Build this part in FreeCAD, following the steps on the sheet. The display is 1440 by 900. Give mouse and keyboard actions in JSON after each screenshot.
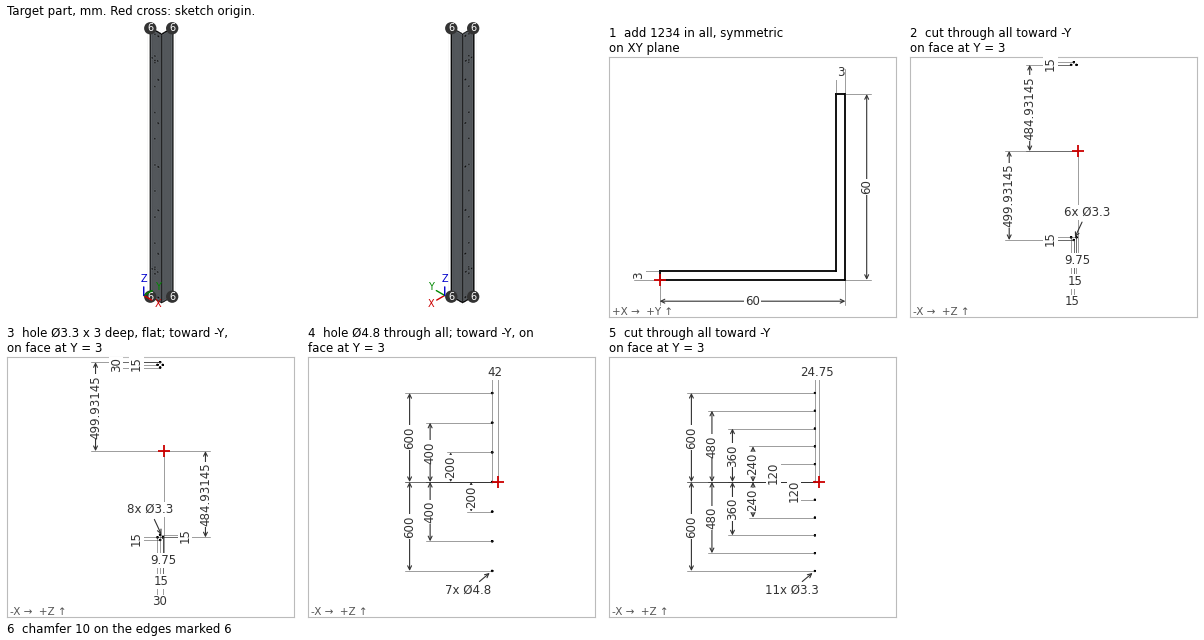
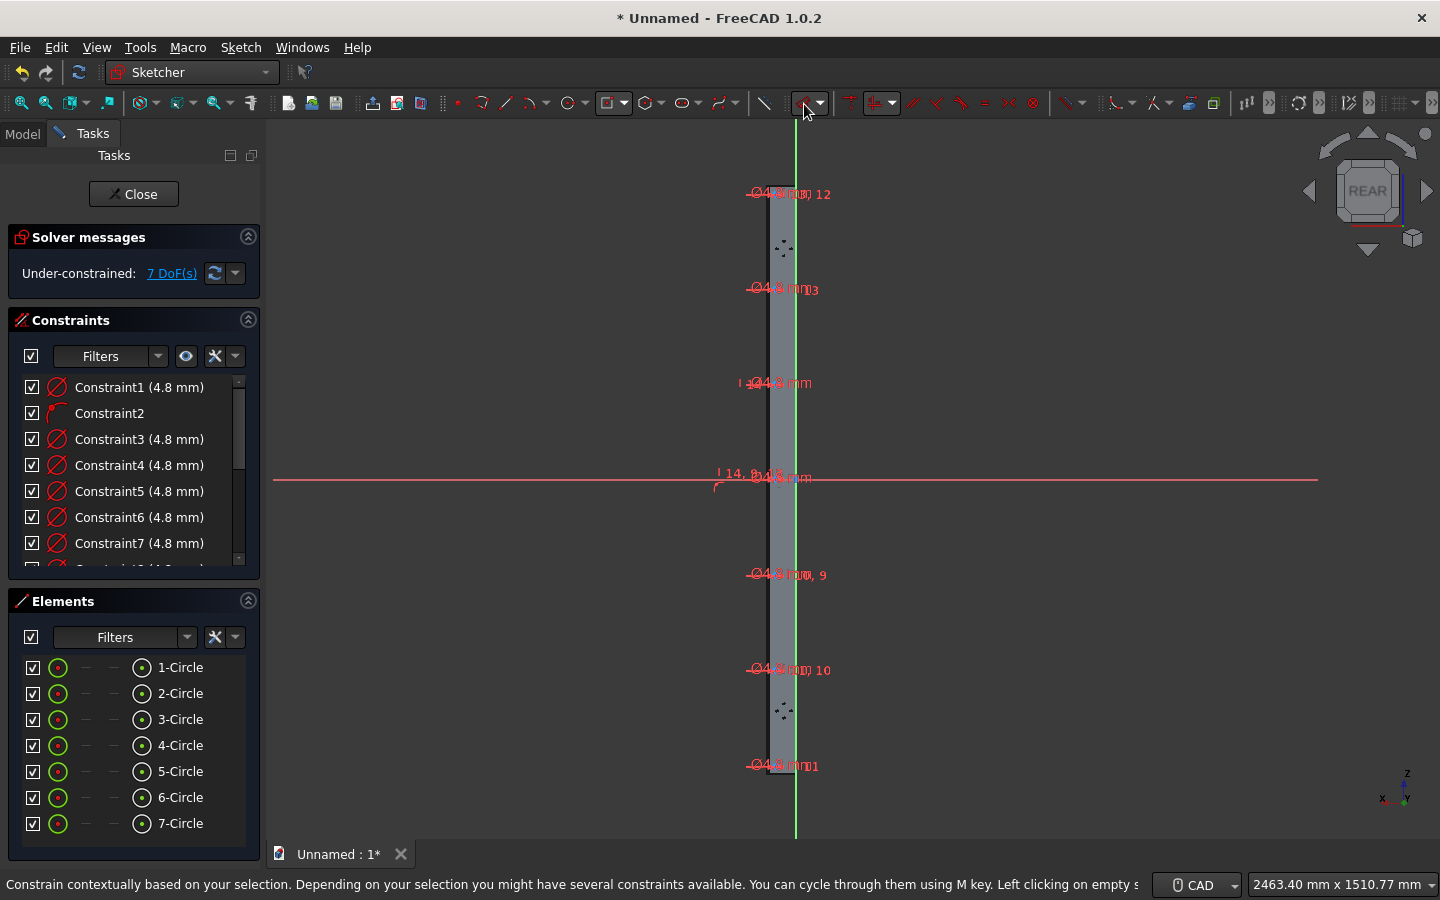
{"action": "scroll", "coordinate": [776, 480], "scroll_direction": "up", "scroll_amount": 4}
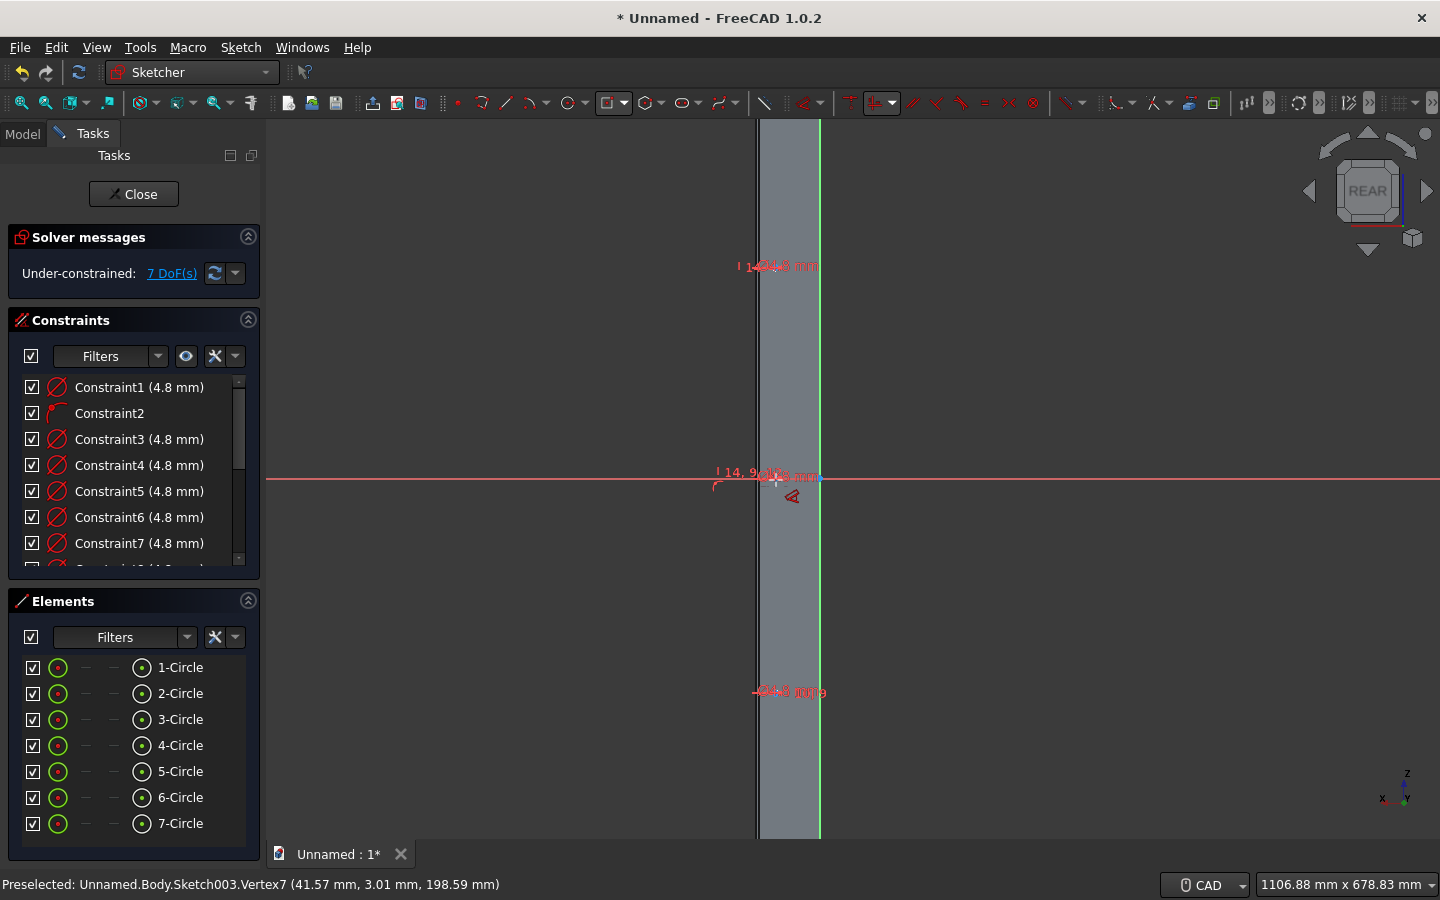
{"action": "left_click", "coordinate": [775, 479]}
{"action": "left_click", "coordinate": [798, 513]}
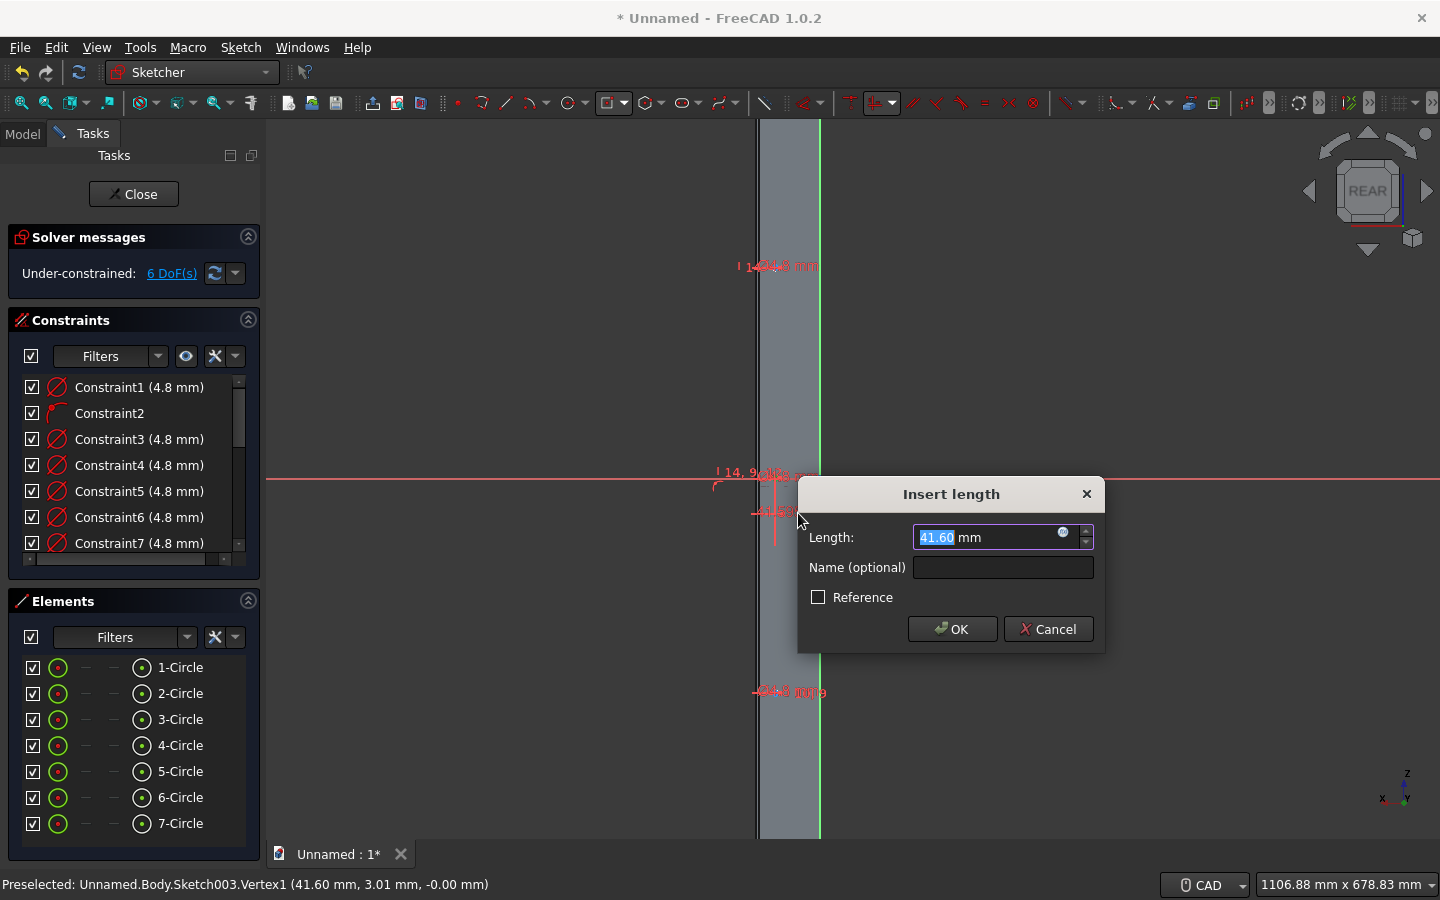
{"action": "type", "text": "42"}
{"action": "key", "text": "Return"}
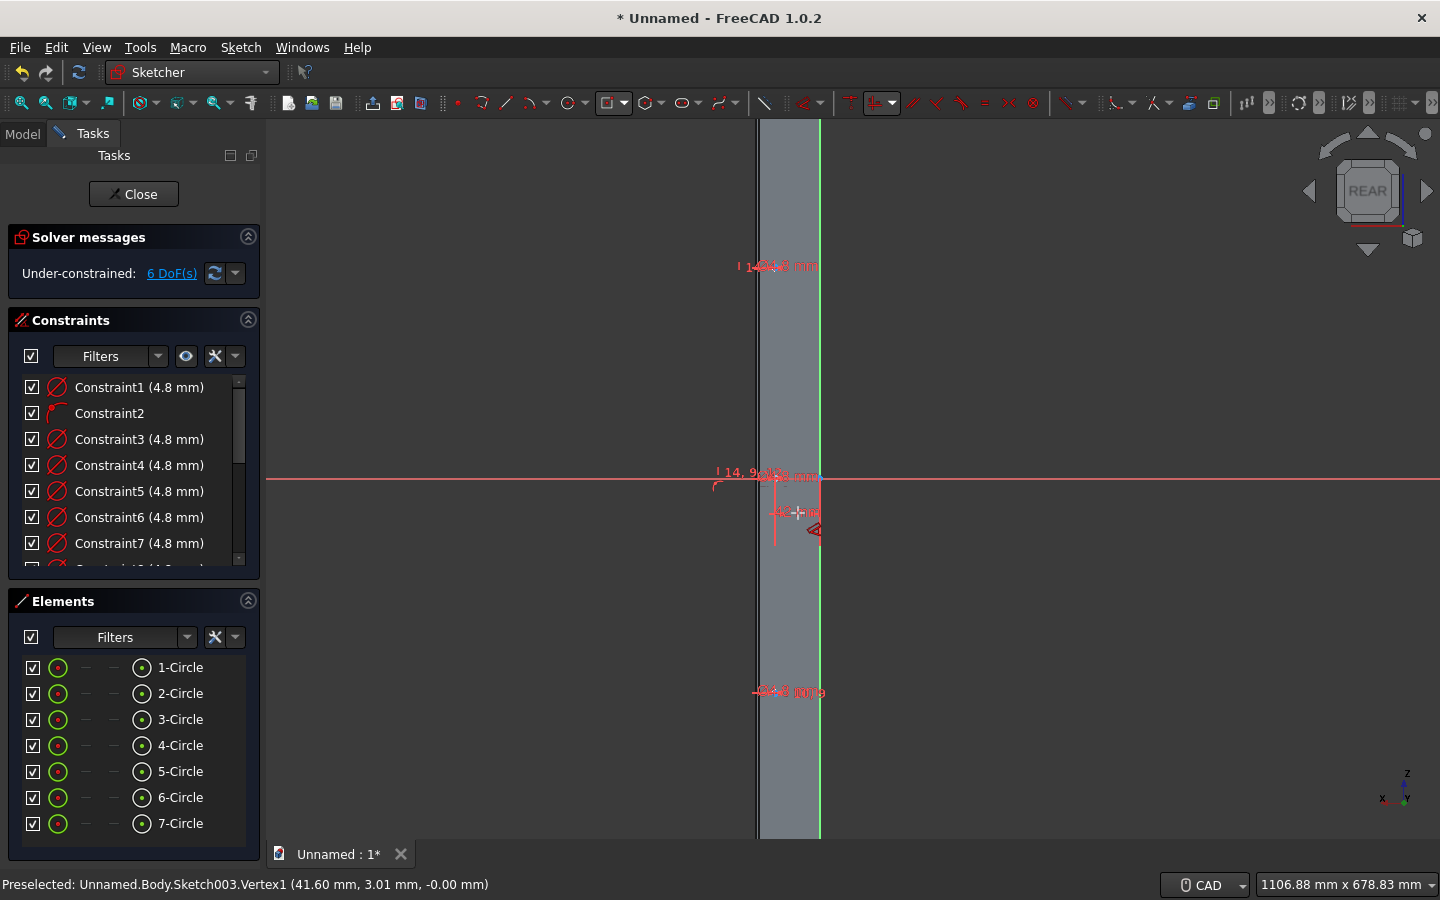
{"action": "left_click", "coordinate": [775, 693]}
{"action": "left_click", "coordinate": [854, 586]}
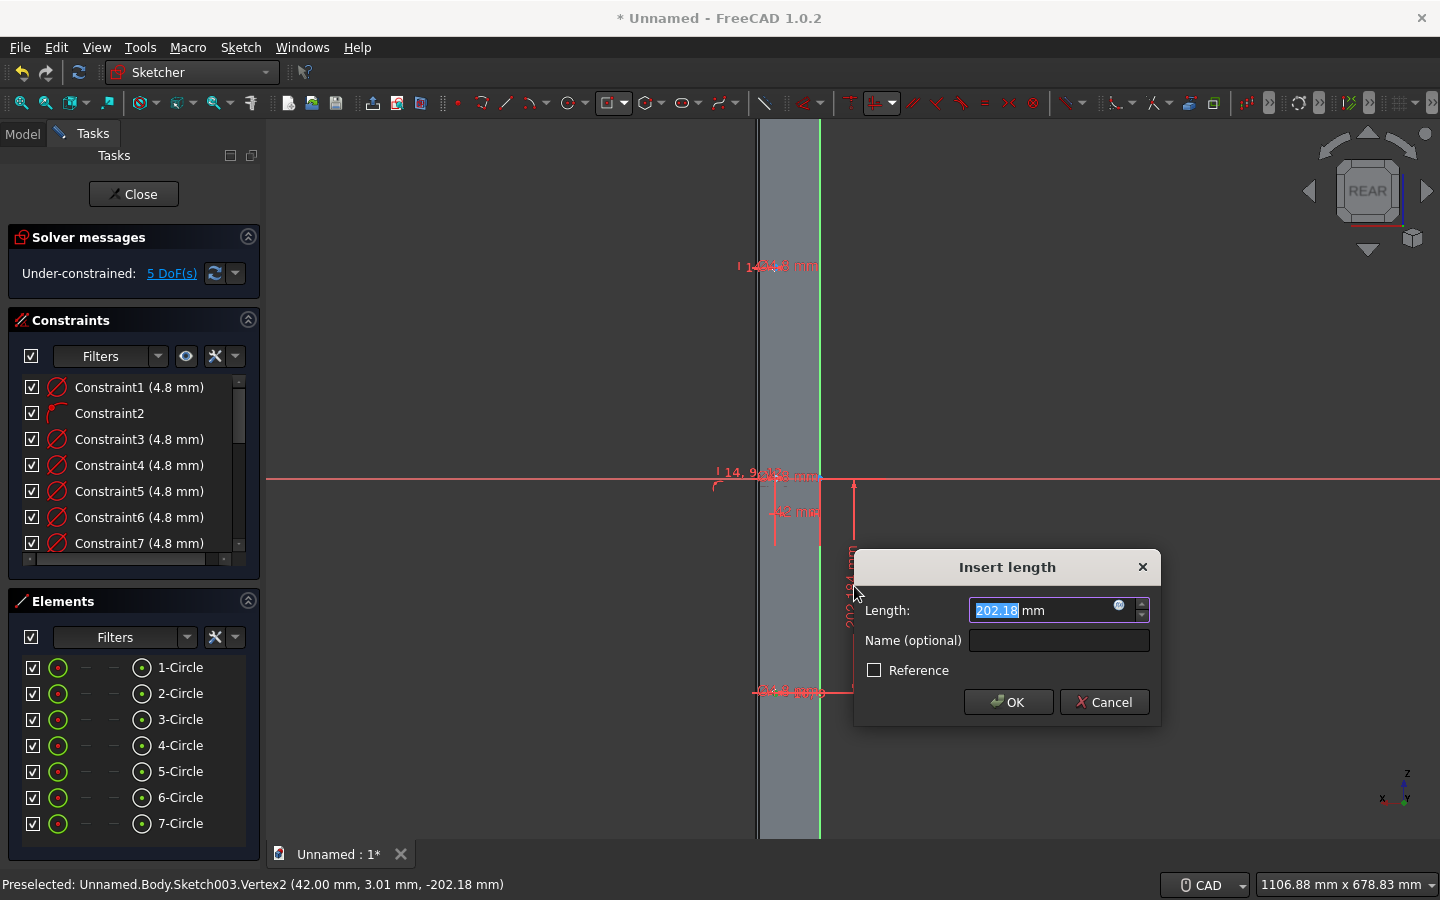
{"action": "type", "text": "200"}
{"action": "key", "text": "Return"}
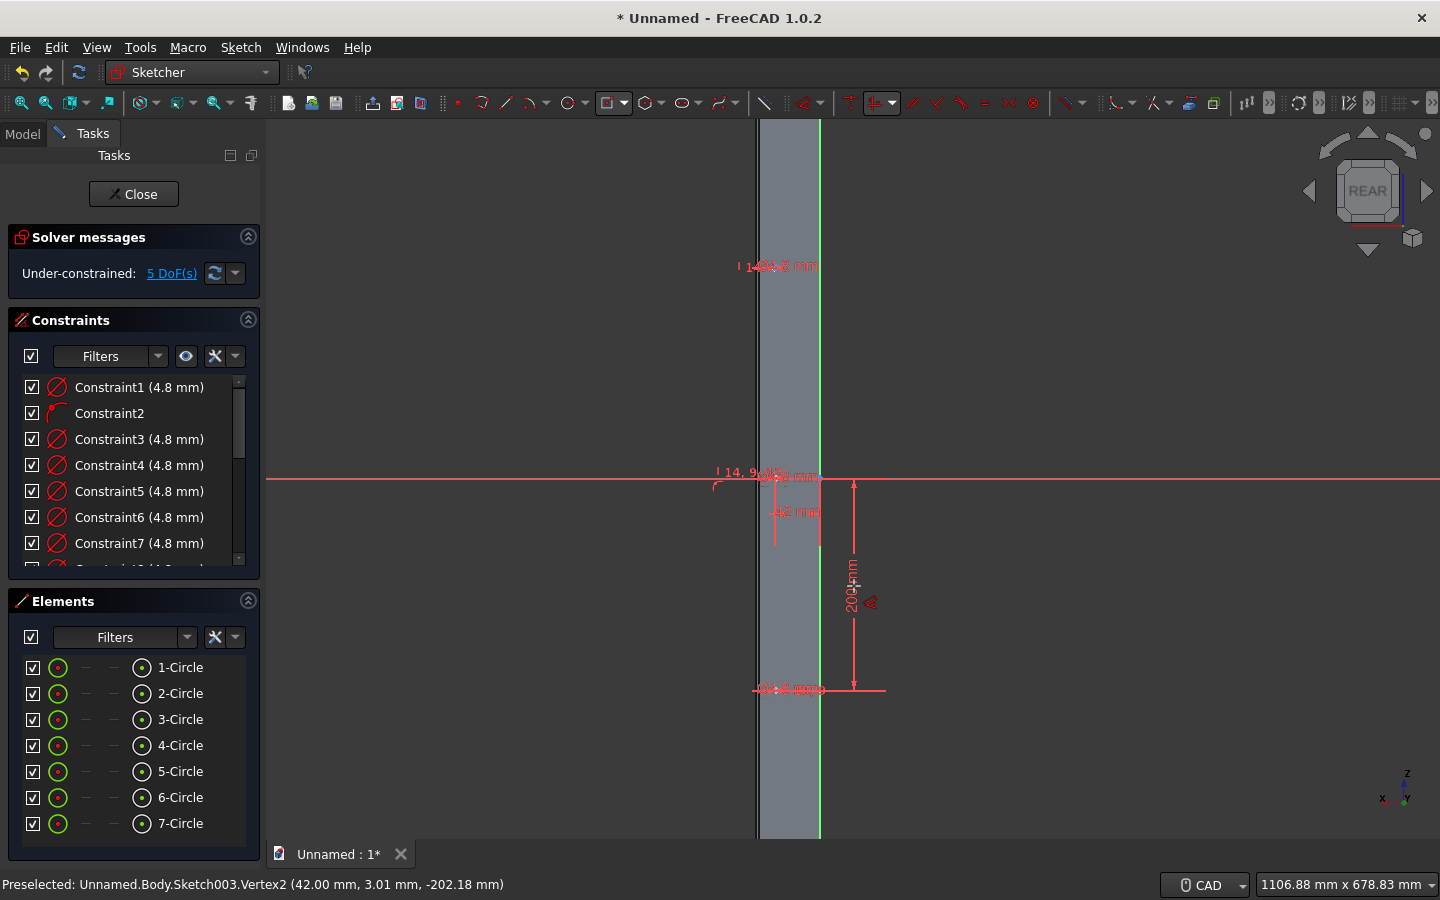
{"action": "scroll", "coordinate": [778, 479], "scroll_direction": "down", "scroll_amount": 5}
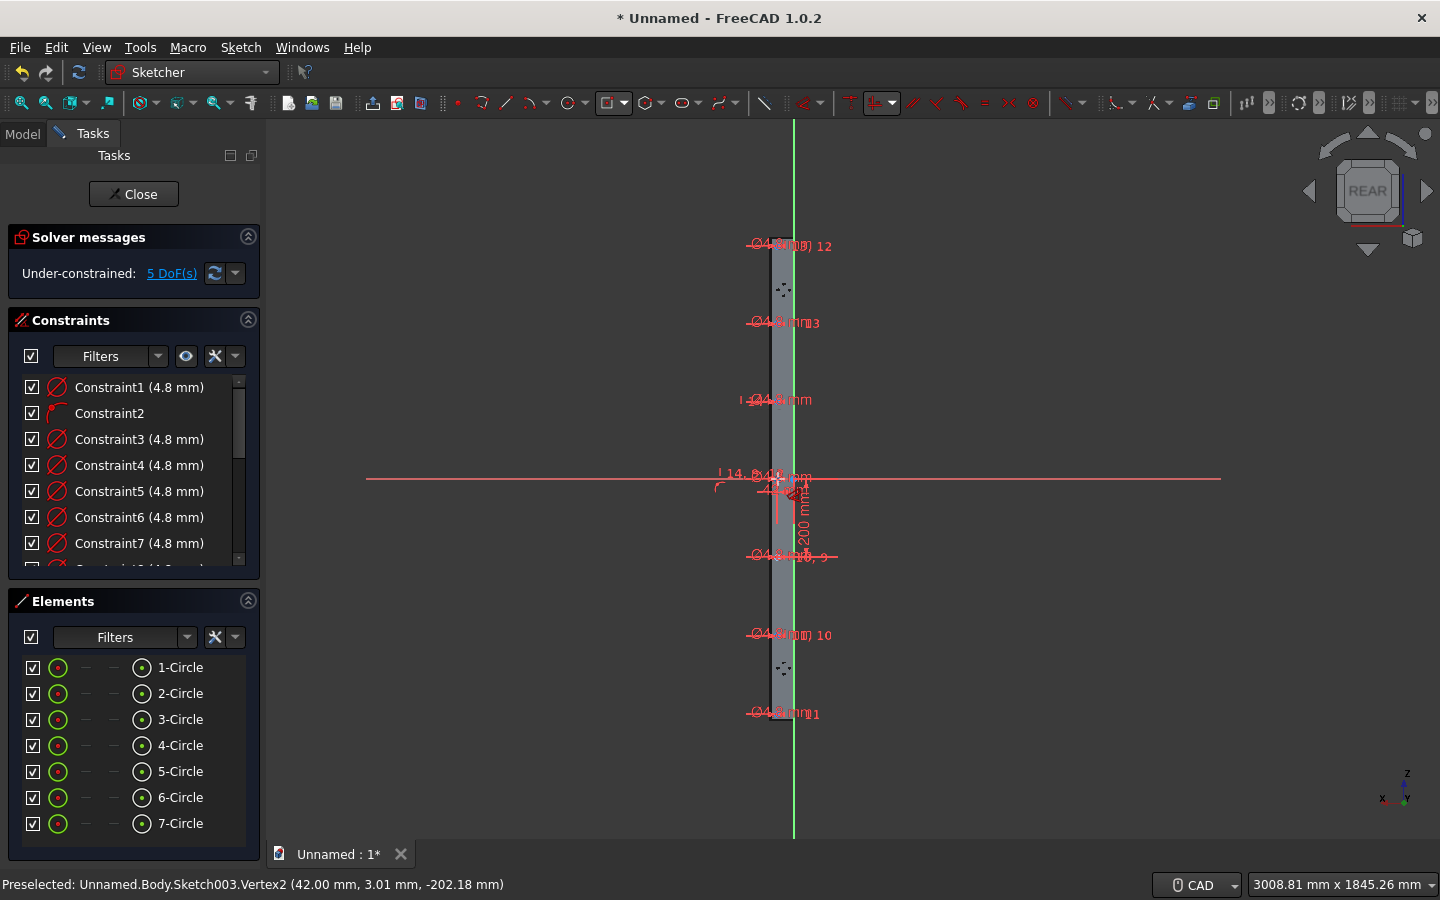
{"action": "left_click", "coordinate": [777, 636]}
{"action": "left_click", "coordinate": [828, 558]}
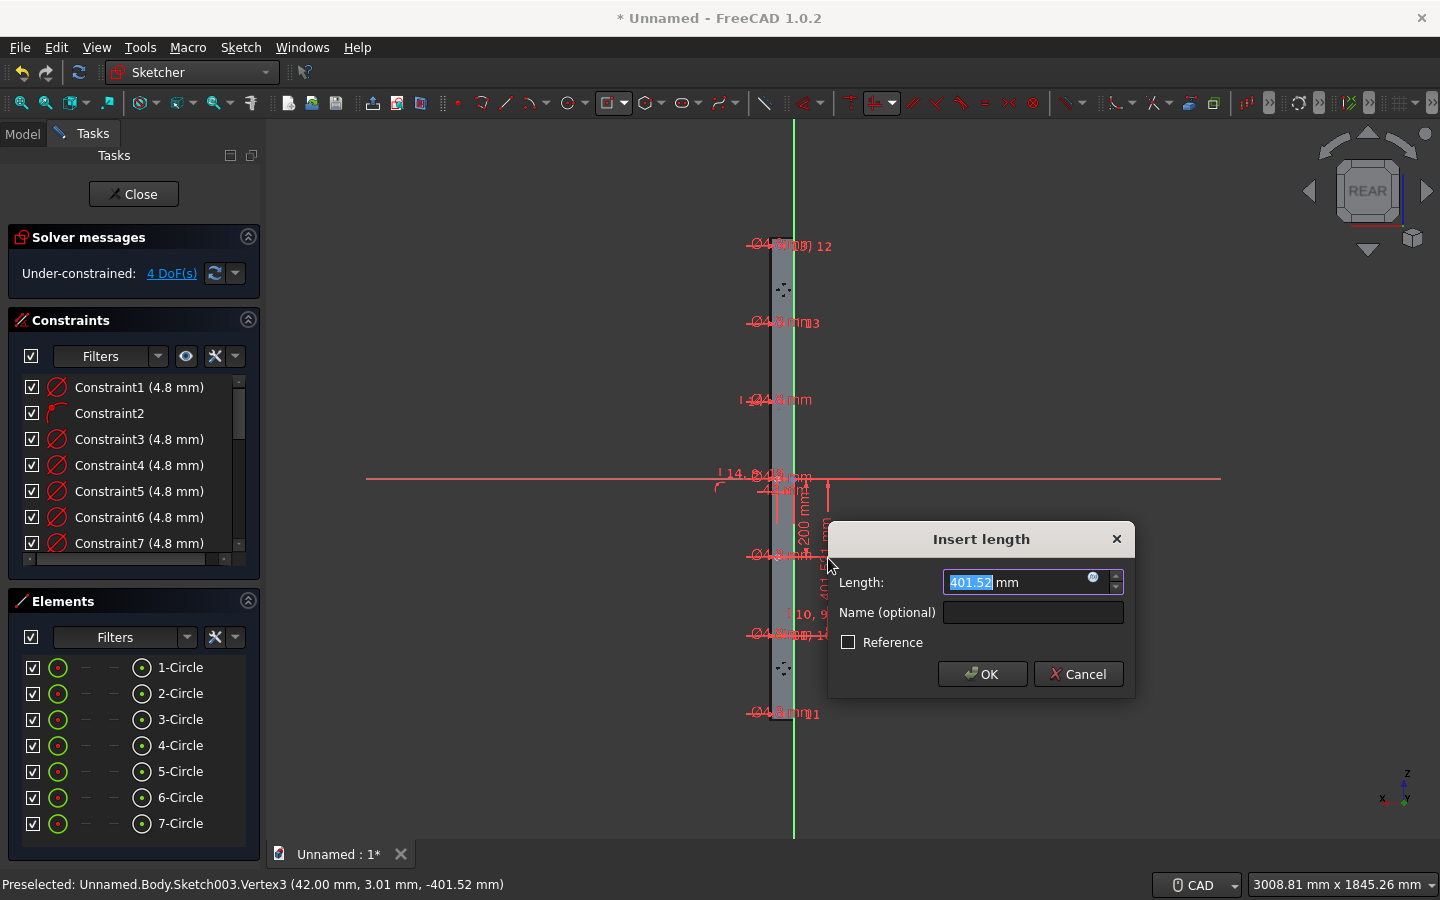
{"action": "type", "text": "400"}
{"action": "key", "text": "Return"}